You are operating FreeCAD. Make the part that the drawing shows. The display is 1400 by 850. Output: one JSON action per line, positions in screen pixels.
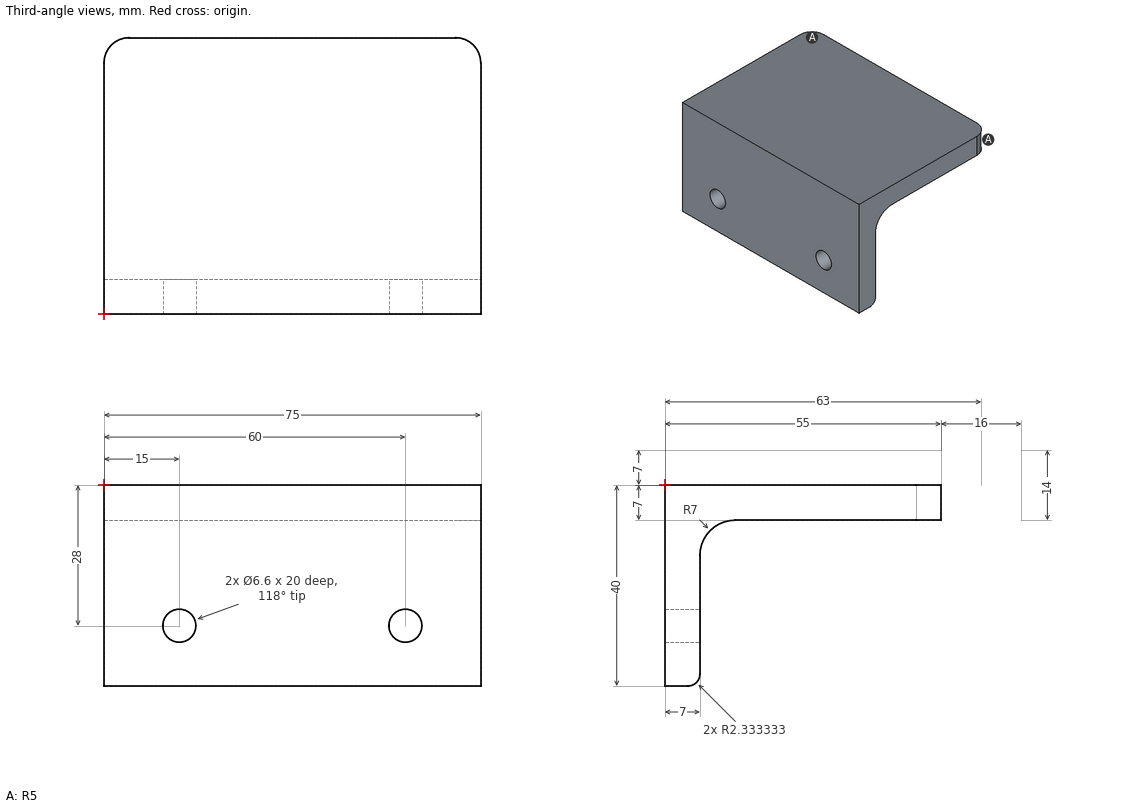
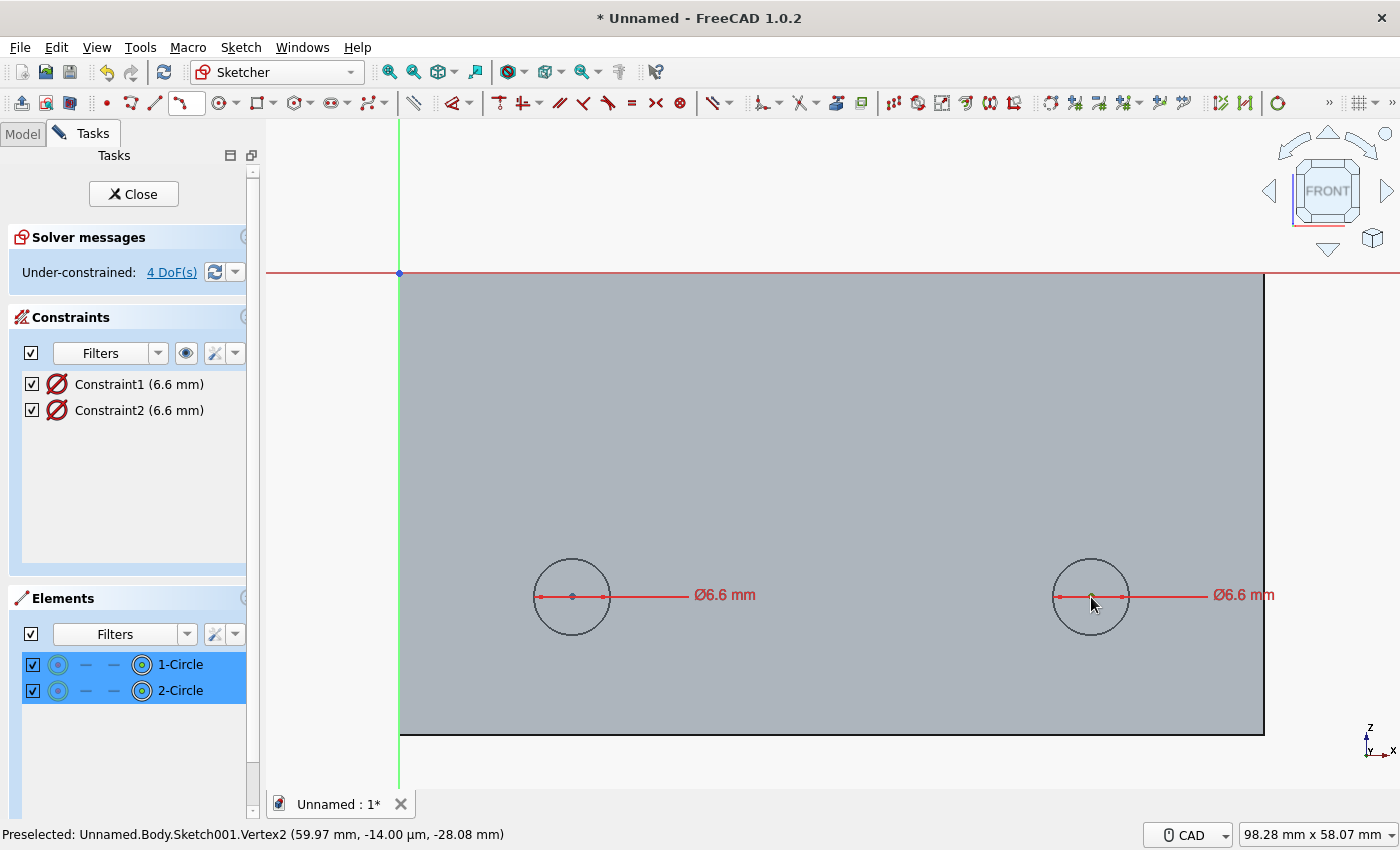
{"action": "key", "text": "h"}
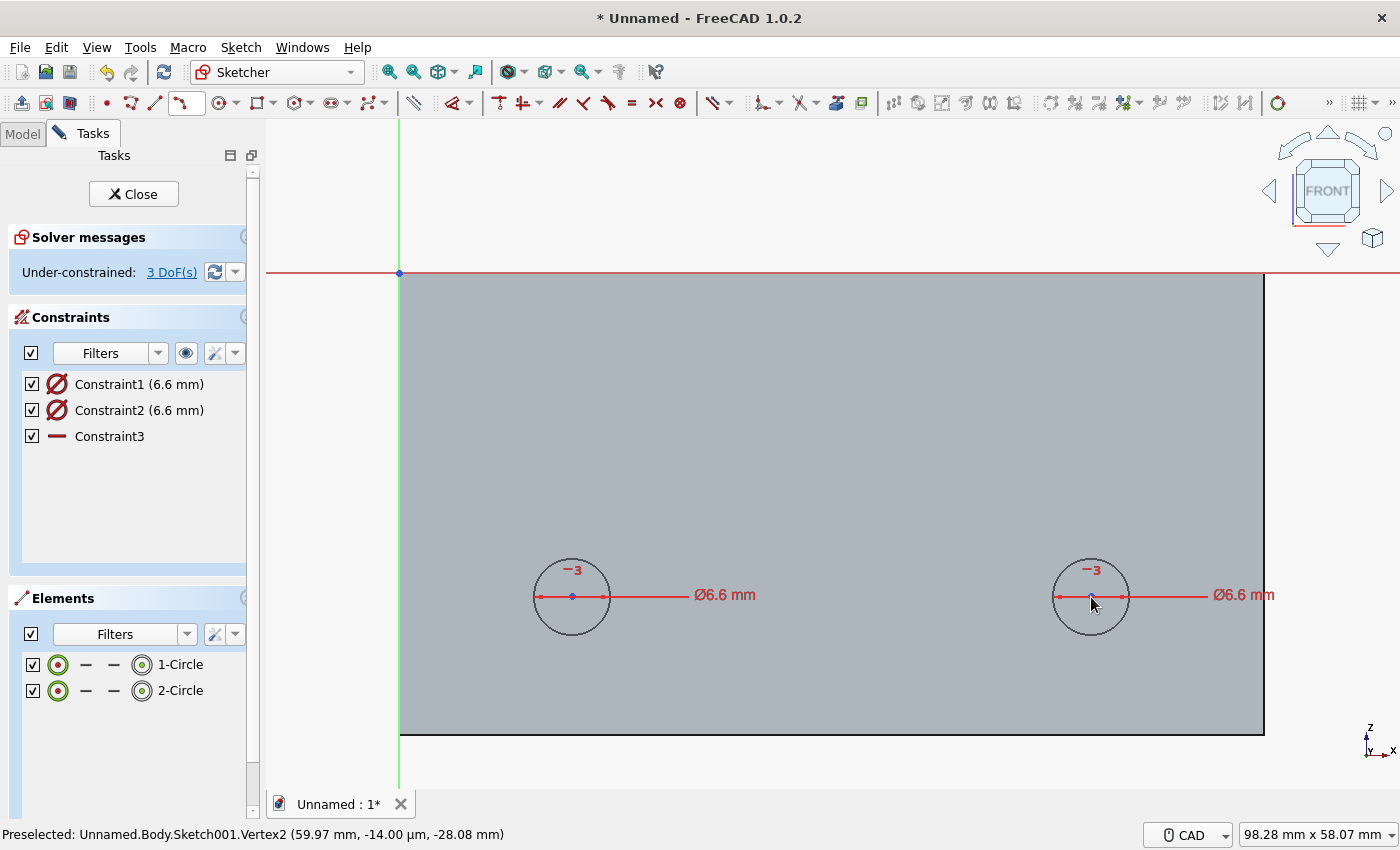
{"action": "left_click", "coordinate": [452, 104]}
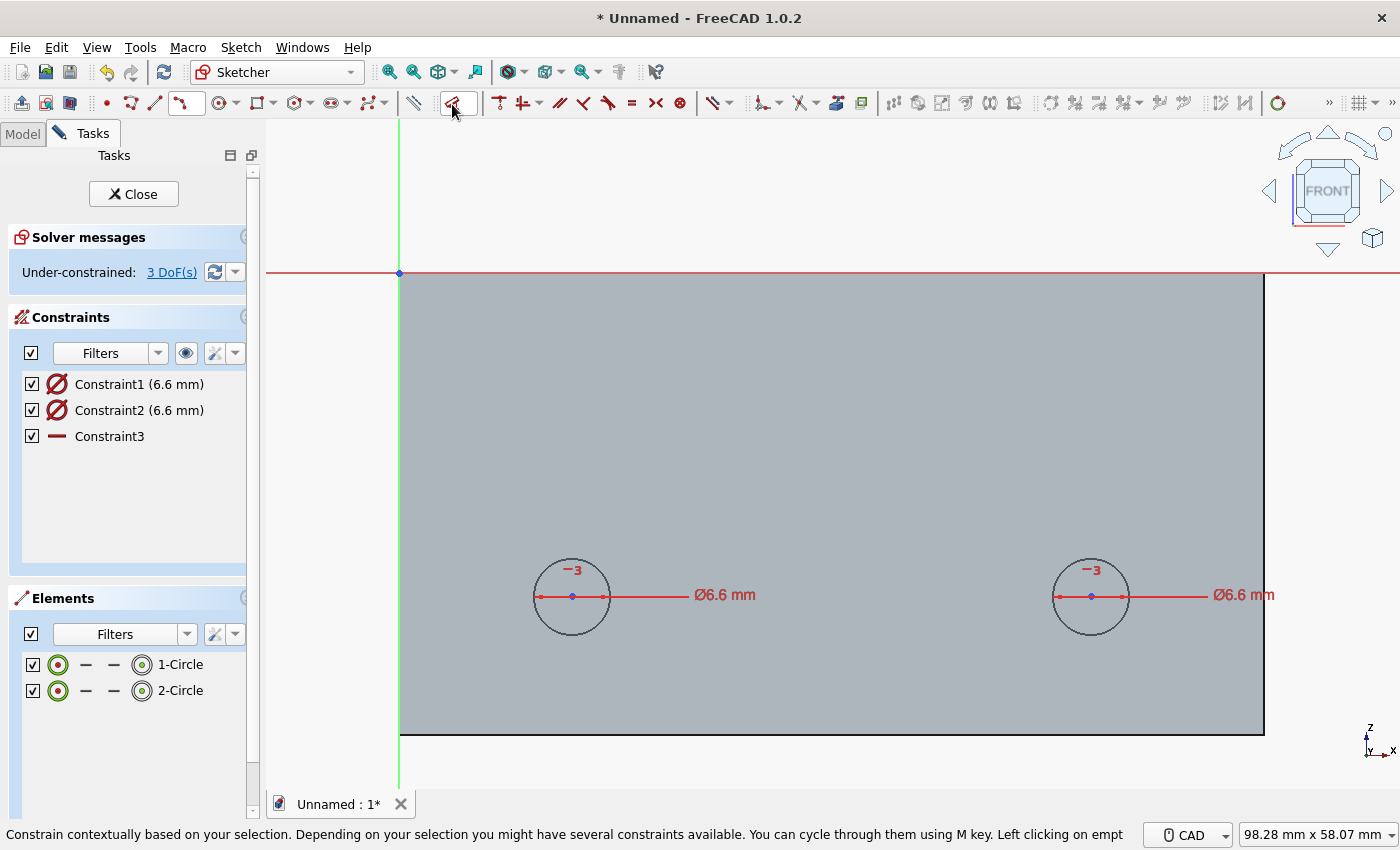
{"action": "left_click", "coordinate": [572, 597]}
{"action": "left_click", "coordinate": [486, 239]}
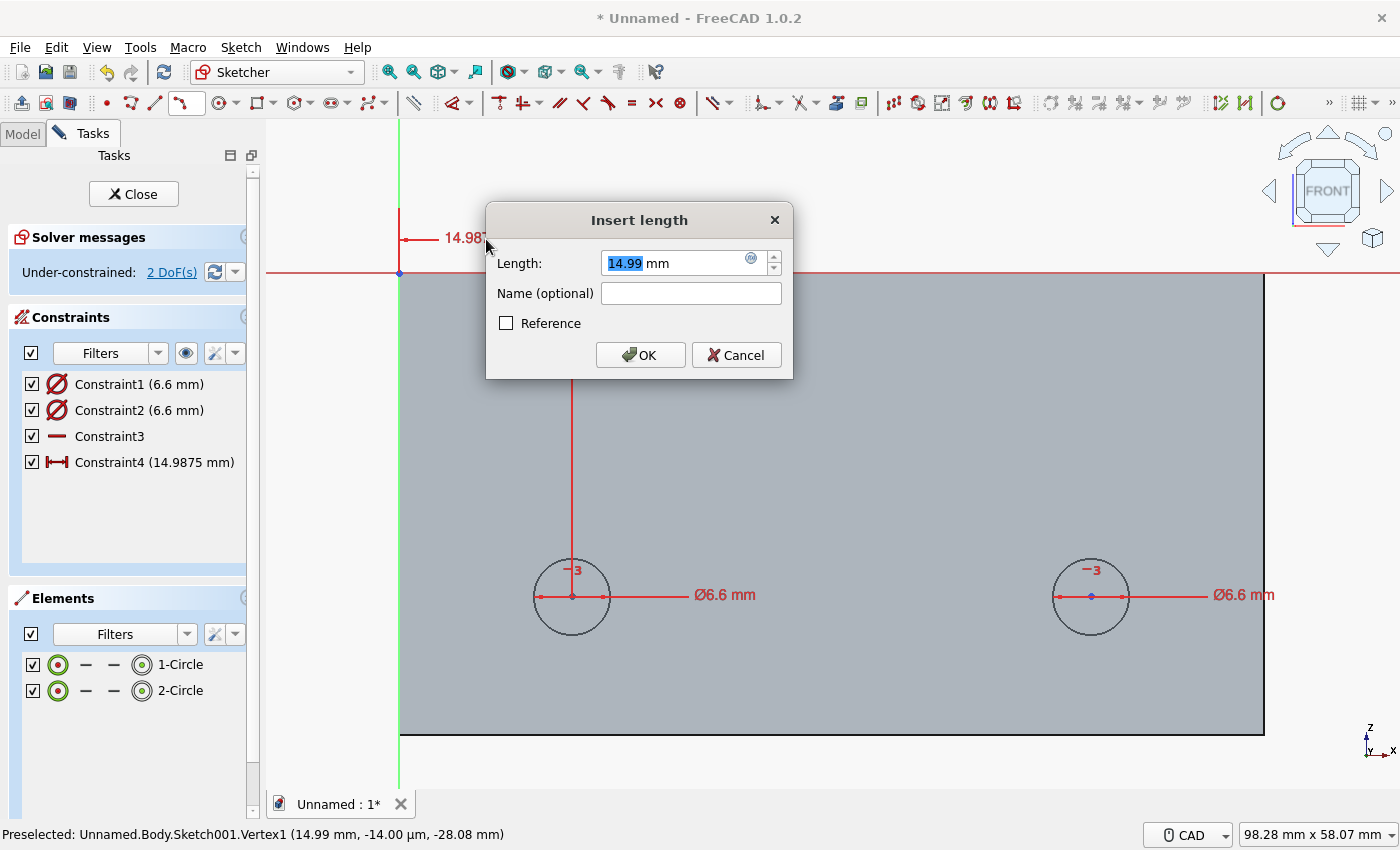
{"action": "type", "text": "15"}
{"action": "key", "text": "Return"}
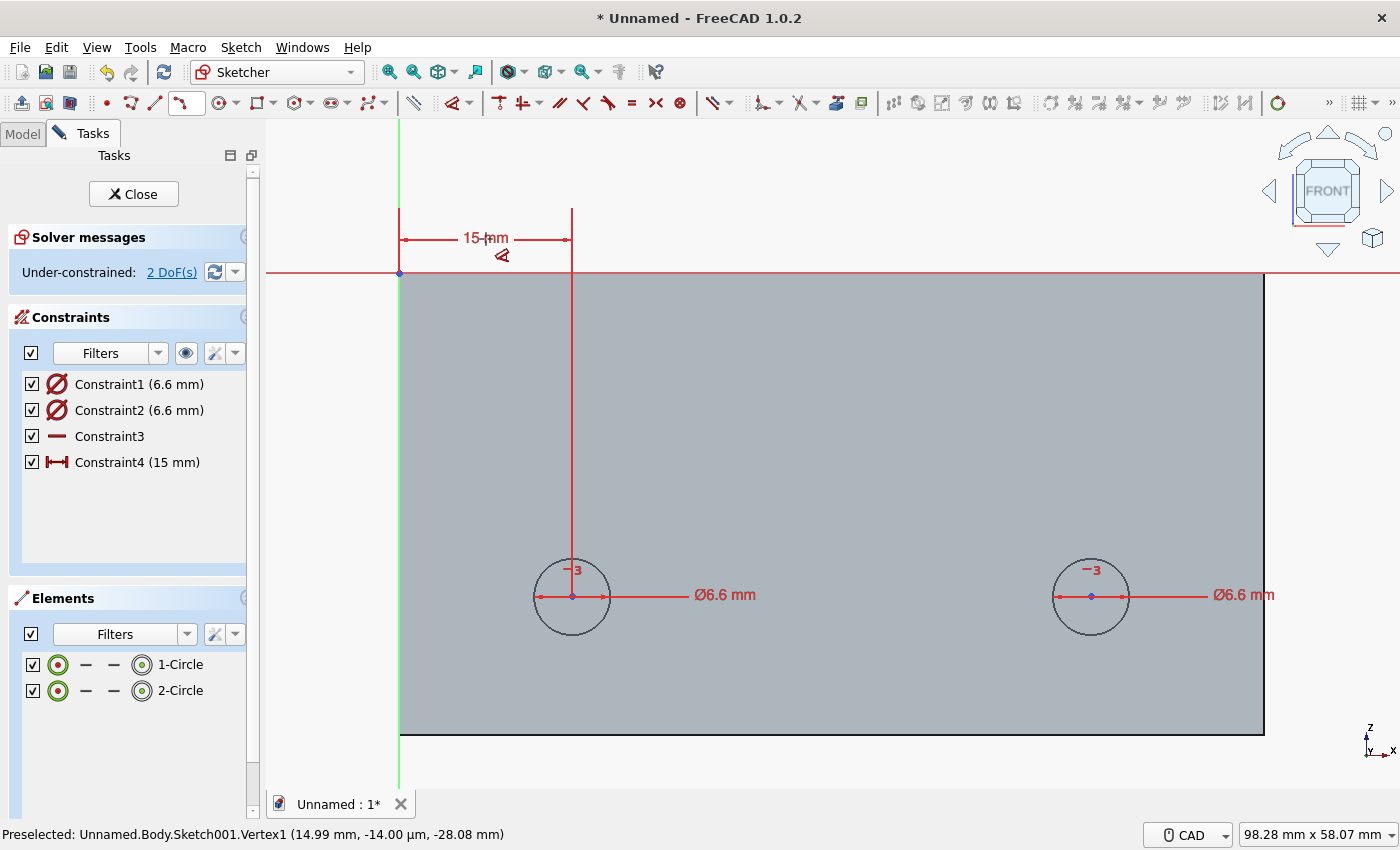
{"action": "left_click", "coordinate": [572, 597]}
{"action": "left_click", "coordinate": [365, 435]}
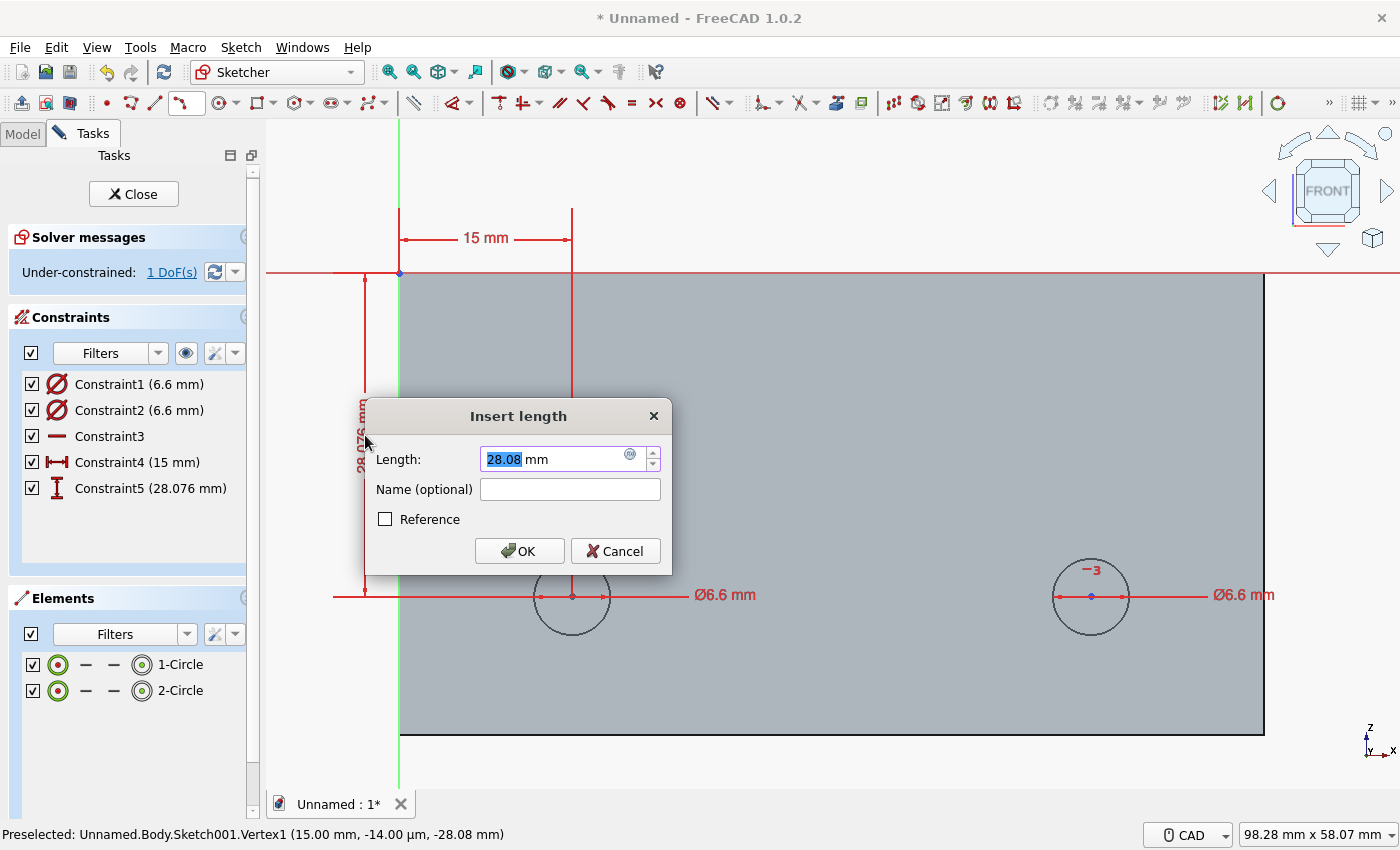
{"action": "type", "text": "28"}
{"action": "key", "text": "Return"}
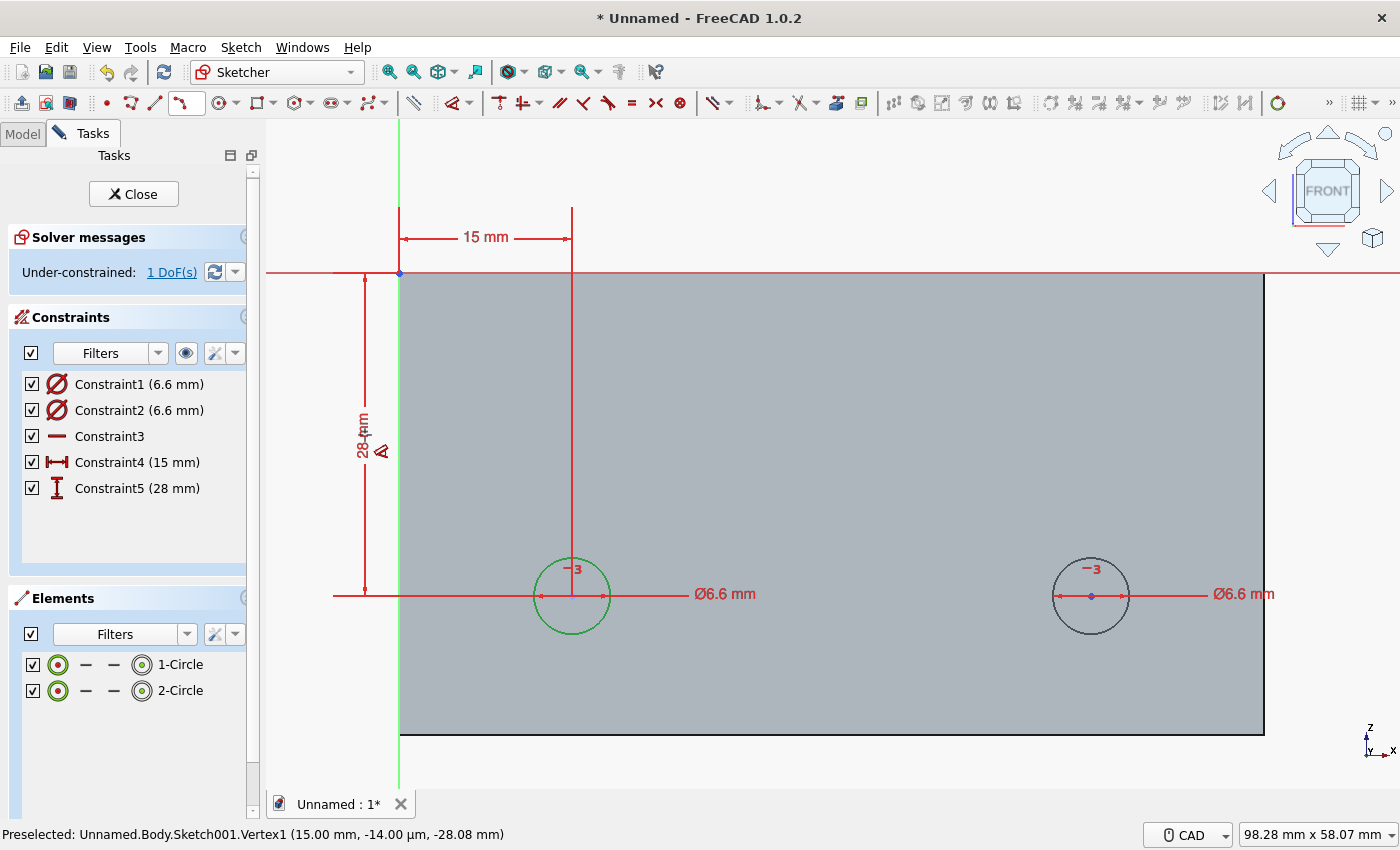
{"action": "left_click", "coordinate": [1091, 596]}
{"action": "left_click", "coordinate": [745, 239]}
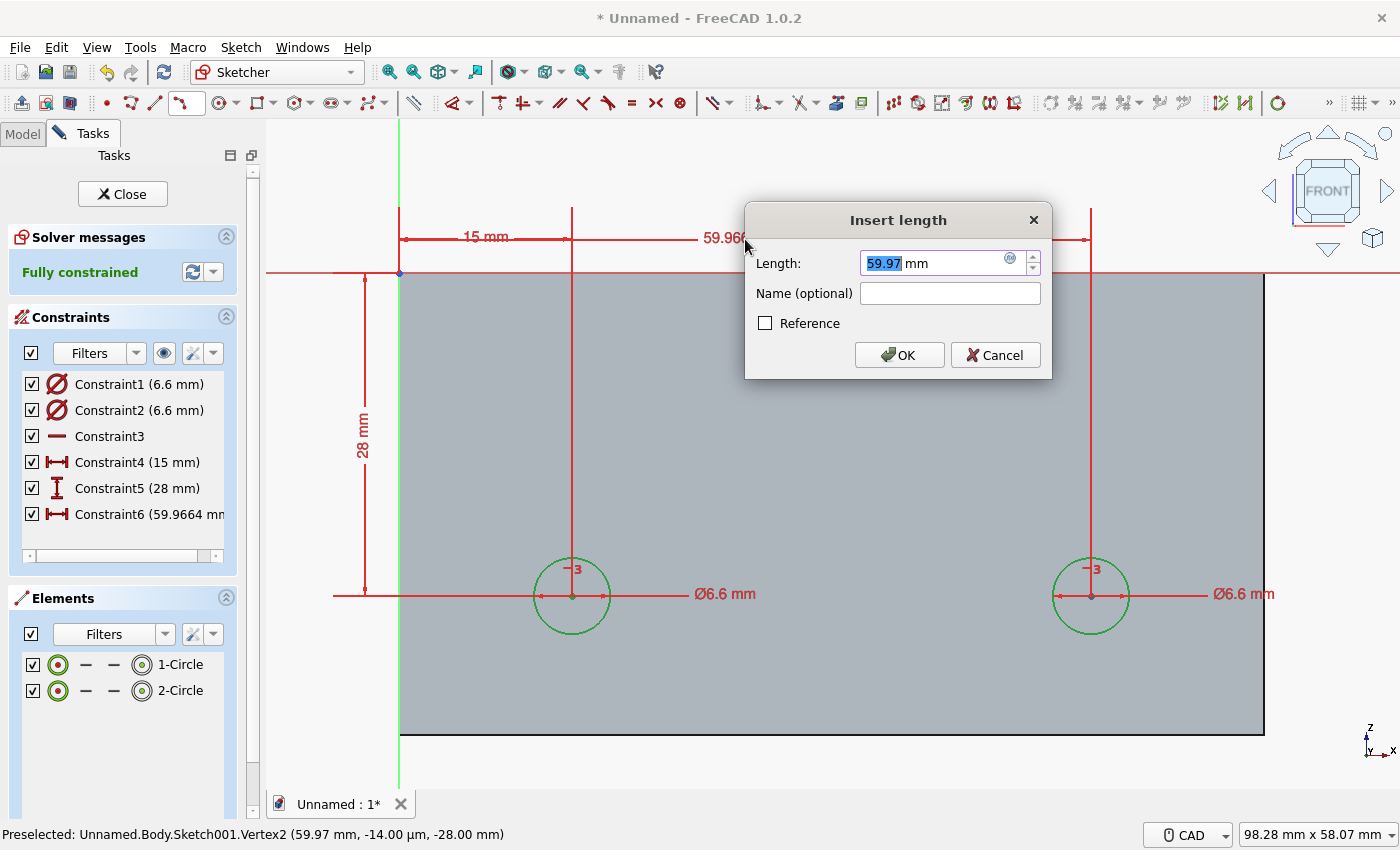
{"action": "type", "text": "60"}
{"action": "key", "text": "Return"}
{"action": "key", "text": "Escape"}